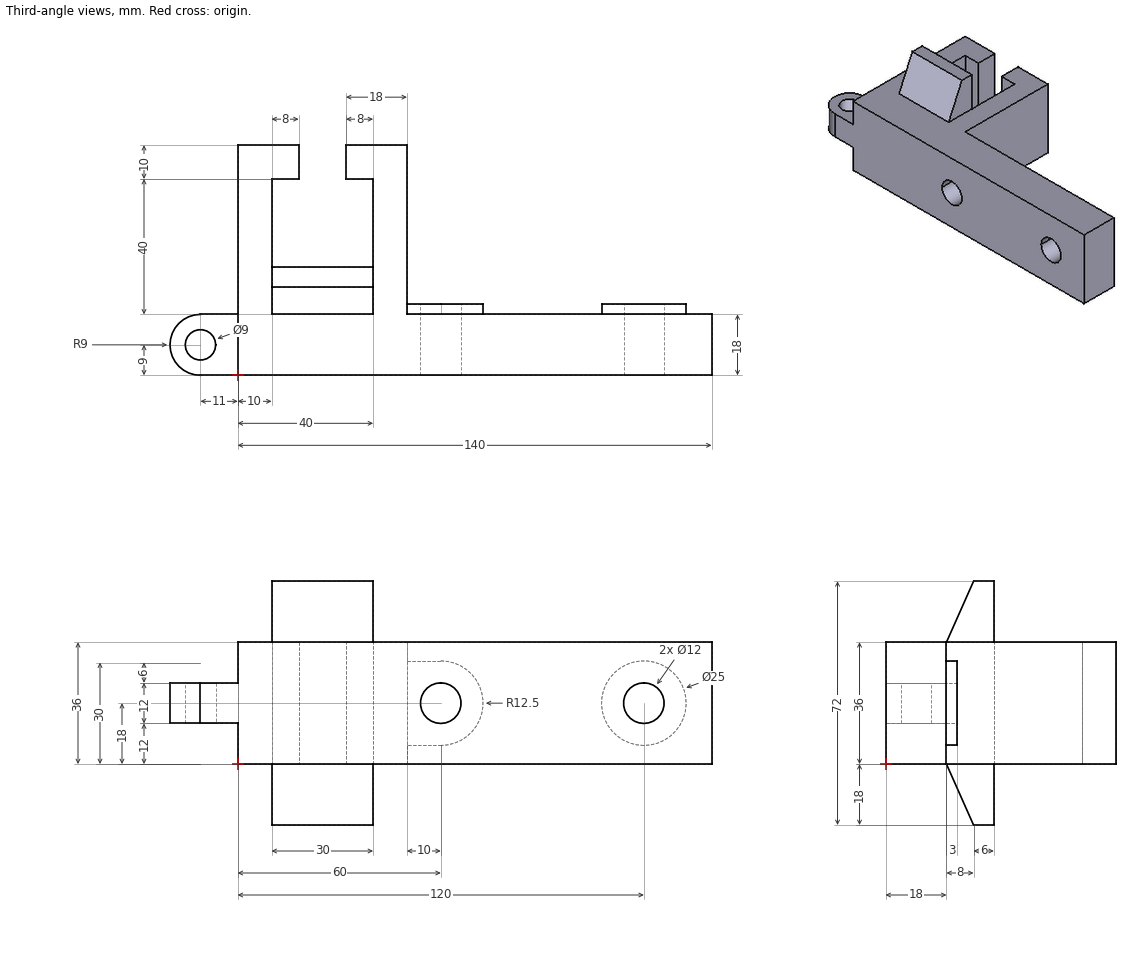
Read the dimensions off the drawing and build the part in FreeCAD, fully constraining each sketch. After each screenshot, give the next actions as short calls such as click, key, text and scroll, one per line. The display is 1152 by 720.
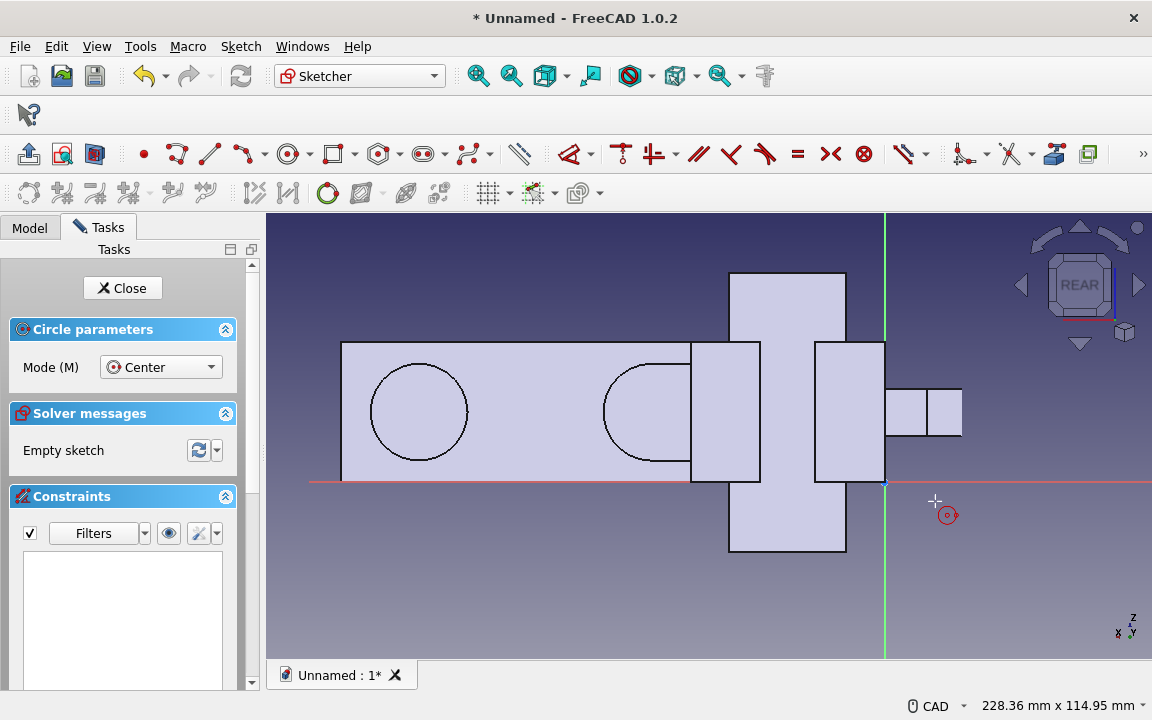
click(419, 412)
click(435, 396)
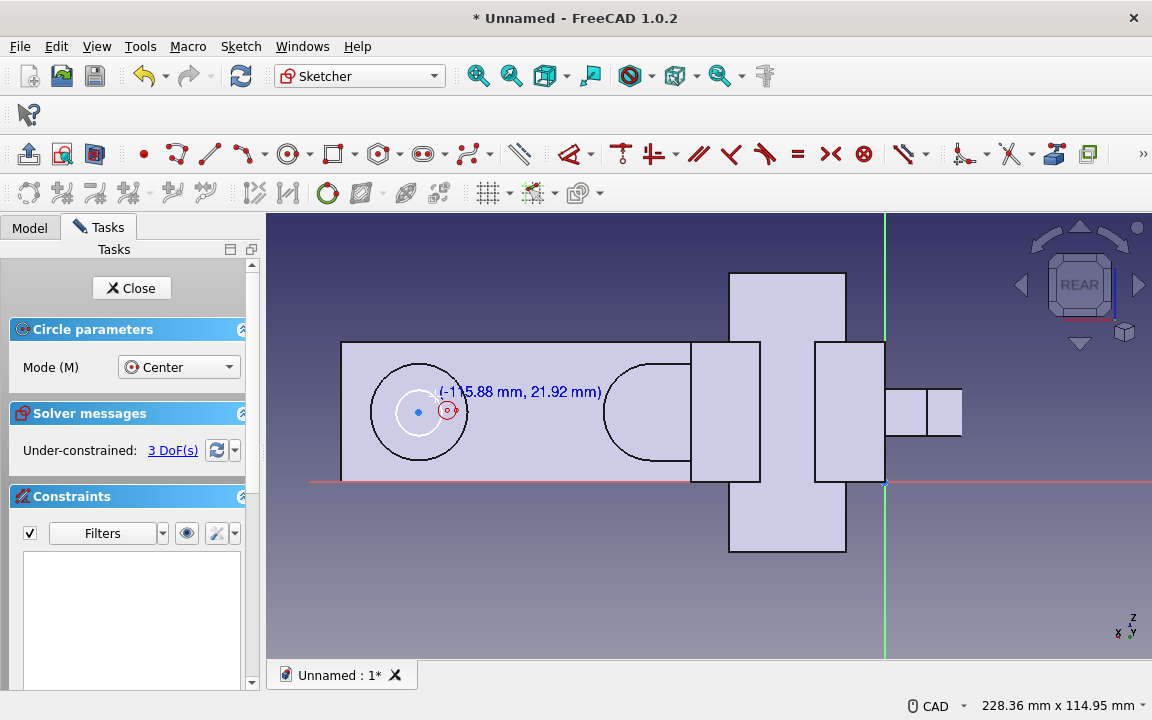
click(652, 412)
click(668, 396)
key(Escape)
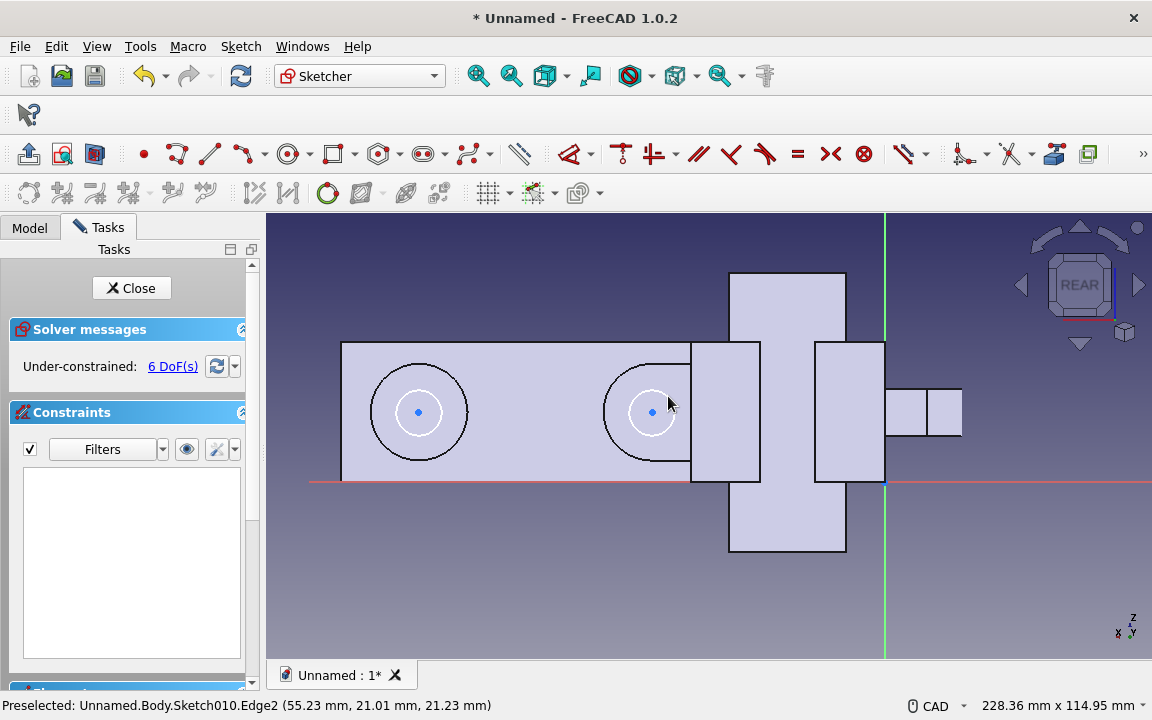
click(435, 397)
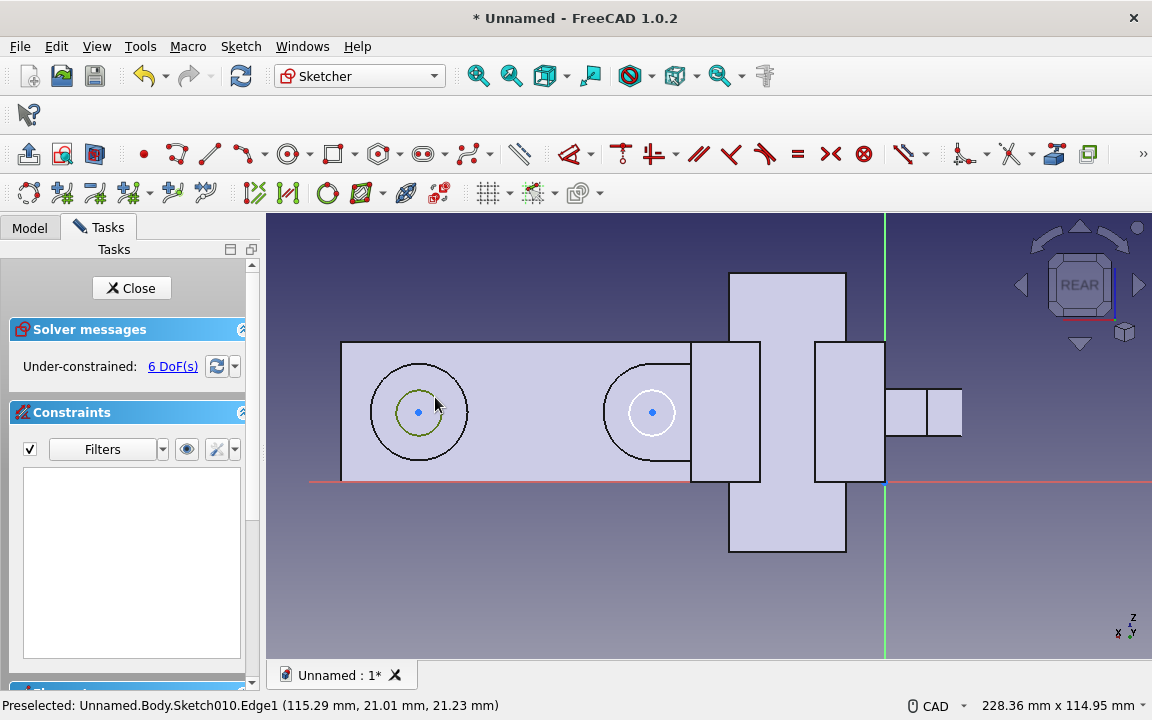
click(668, 397)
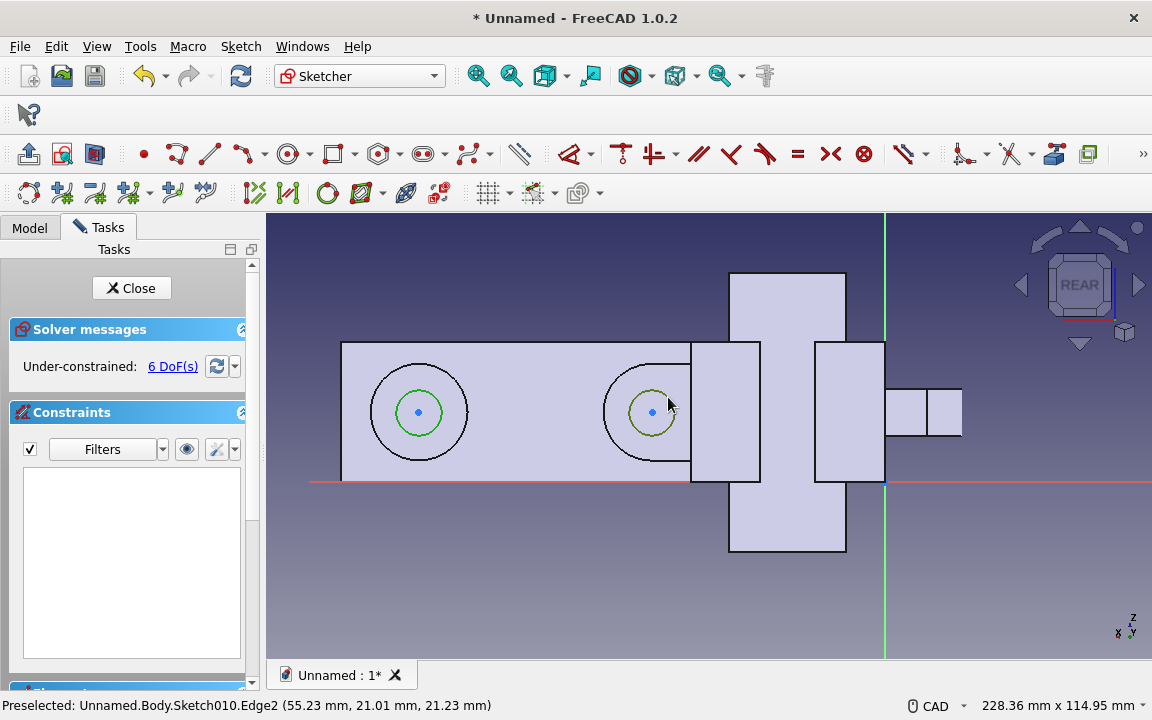
click(798, 154)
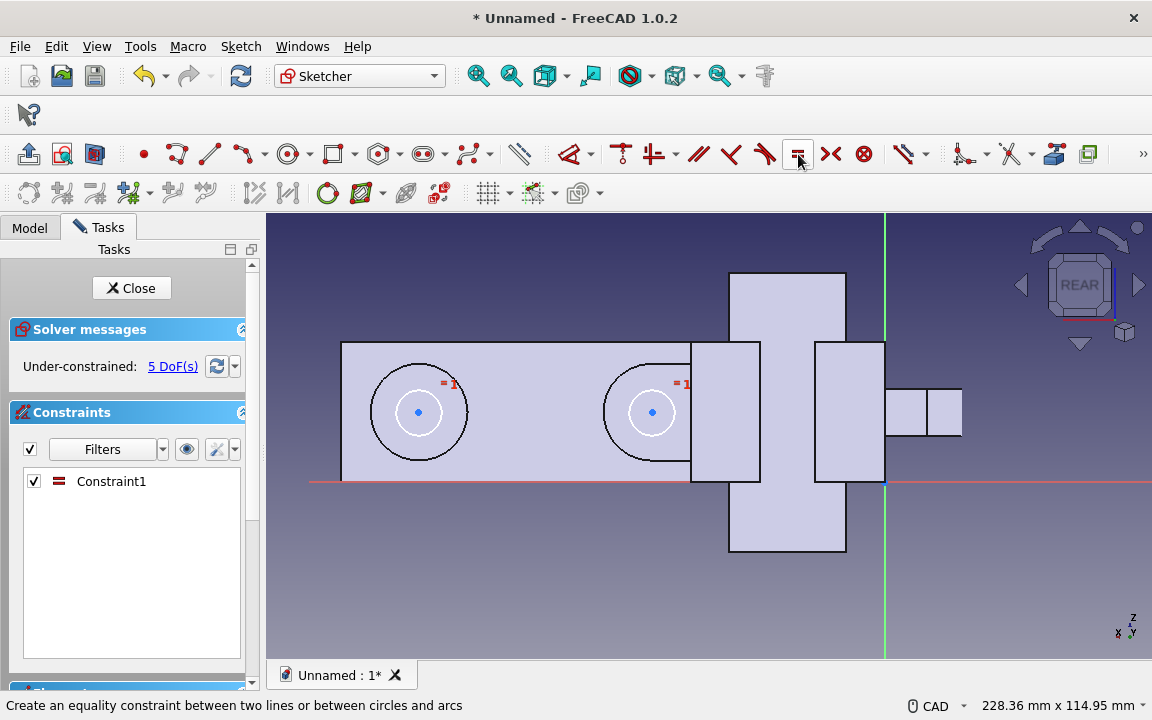
key(d)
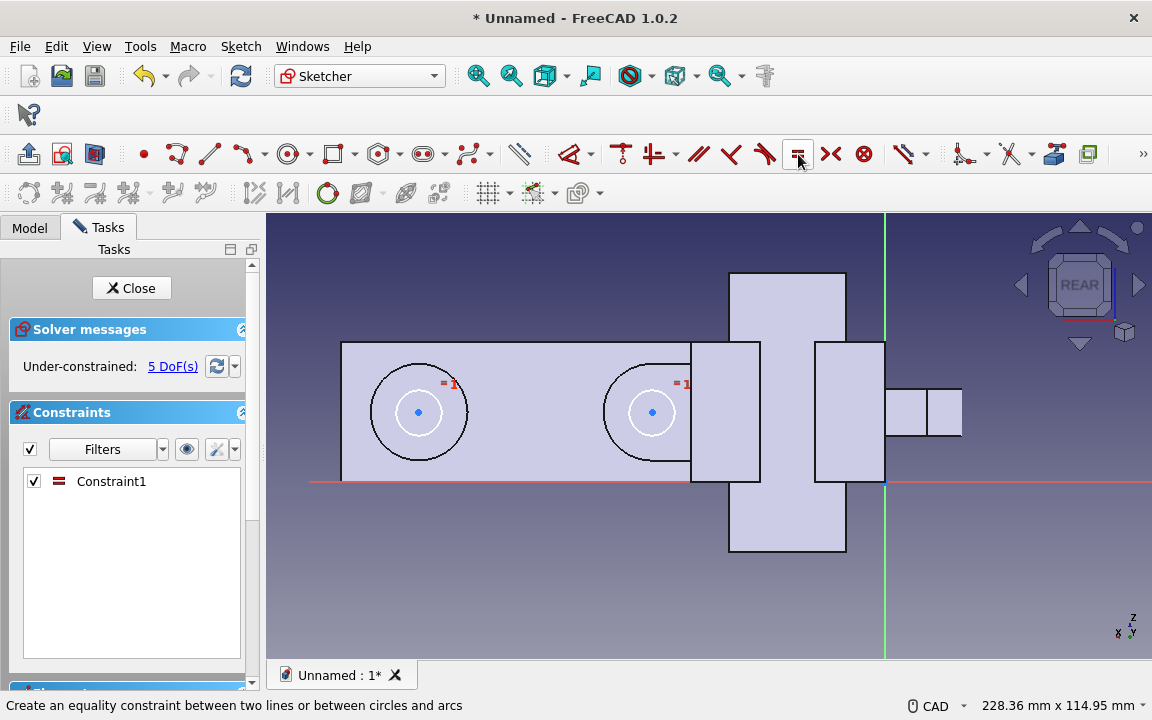
click(435, 397)
click(458, 374)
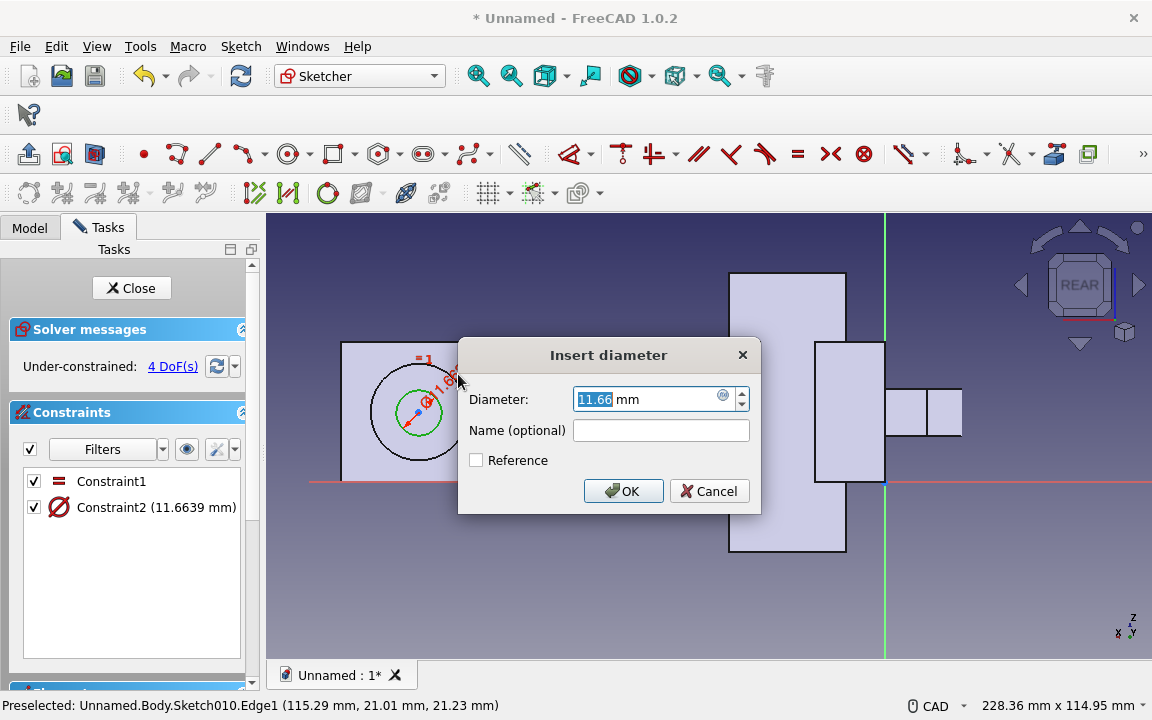
text(12)
key(Return)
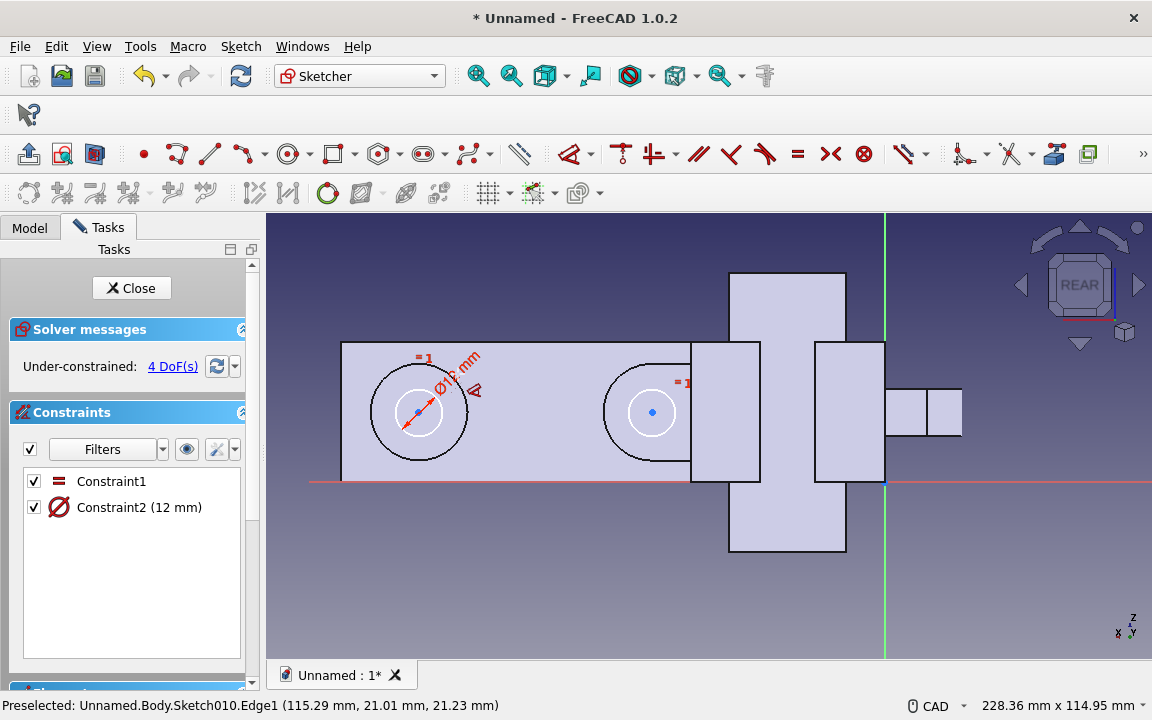
click(419, 413)
click(919, 448)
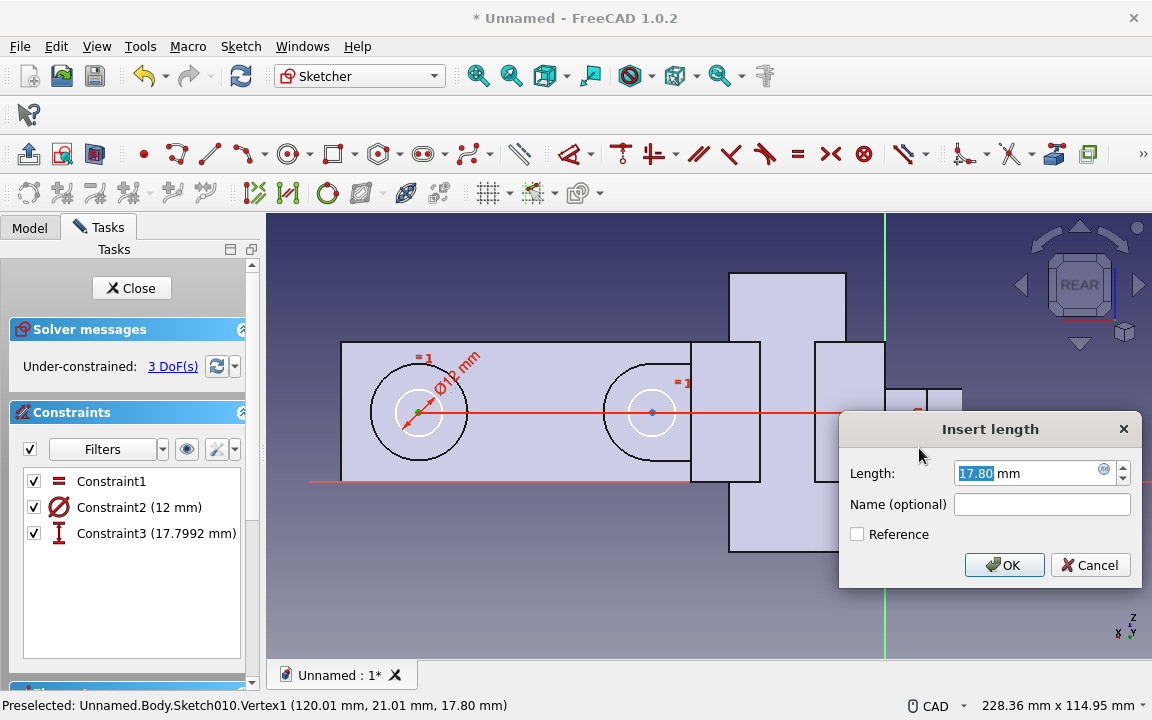
text(18)
key(Return)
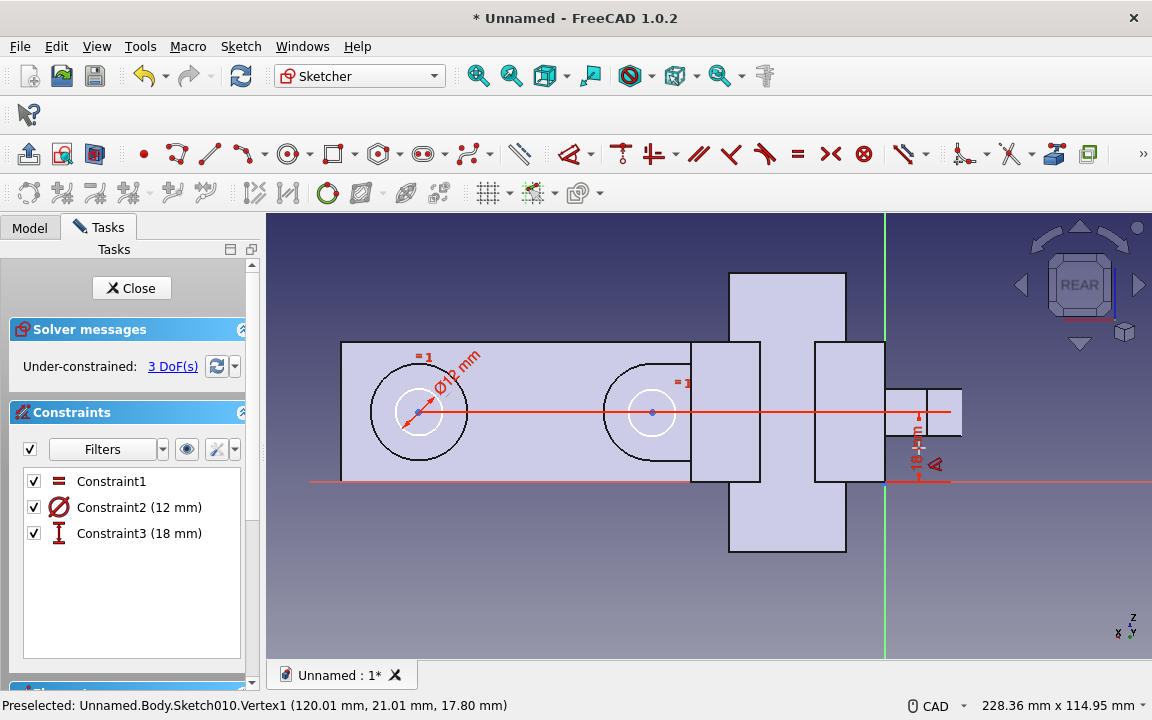
click(652, 413)
click(768, 516)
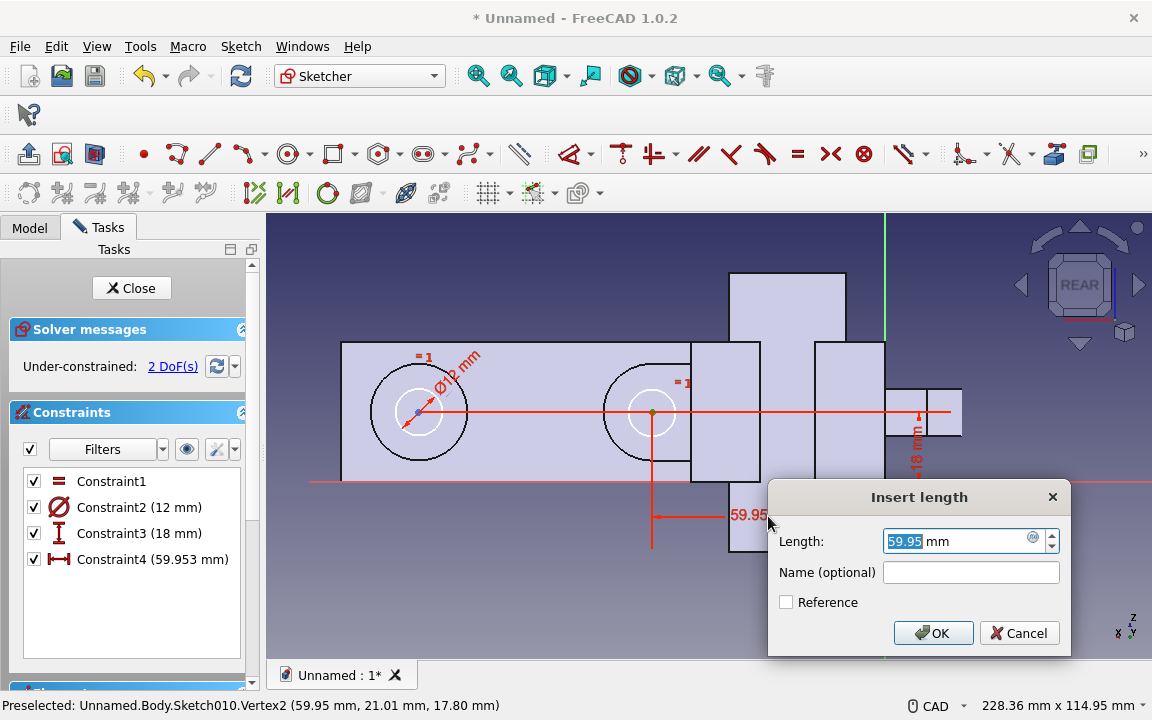
text(60)
key(Return)